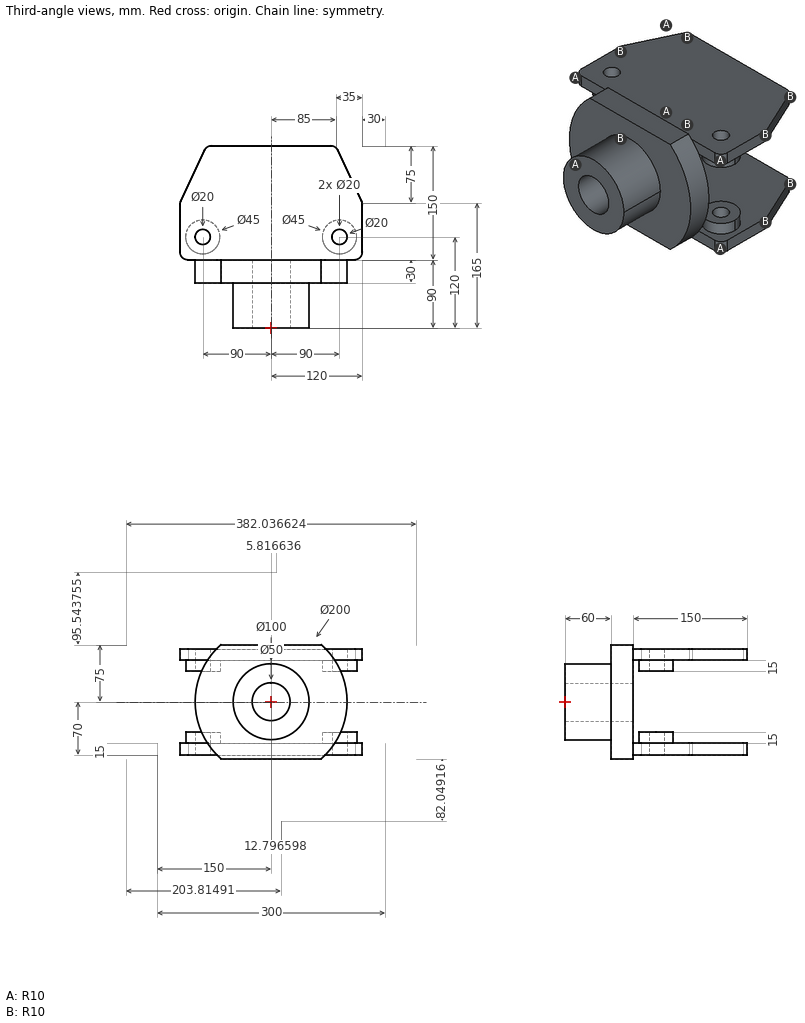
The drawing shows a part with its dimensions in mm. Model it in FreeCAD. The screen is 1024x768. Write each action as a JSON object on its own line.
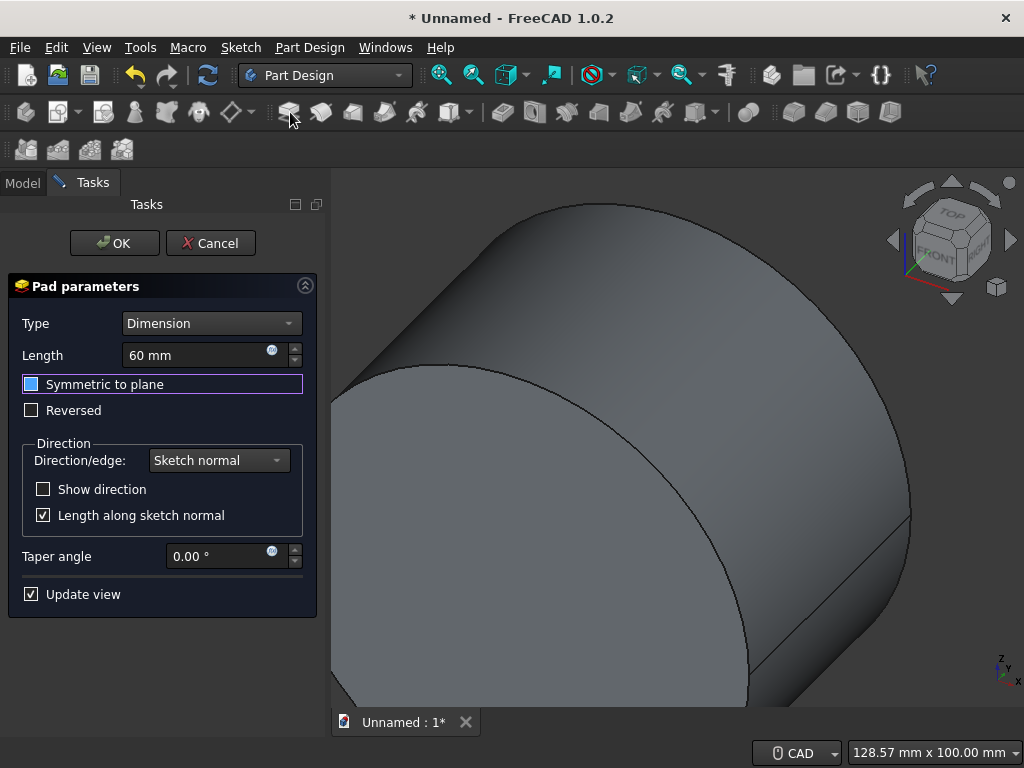
{"action": "left_click", "coordinate": [30, 410]}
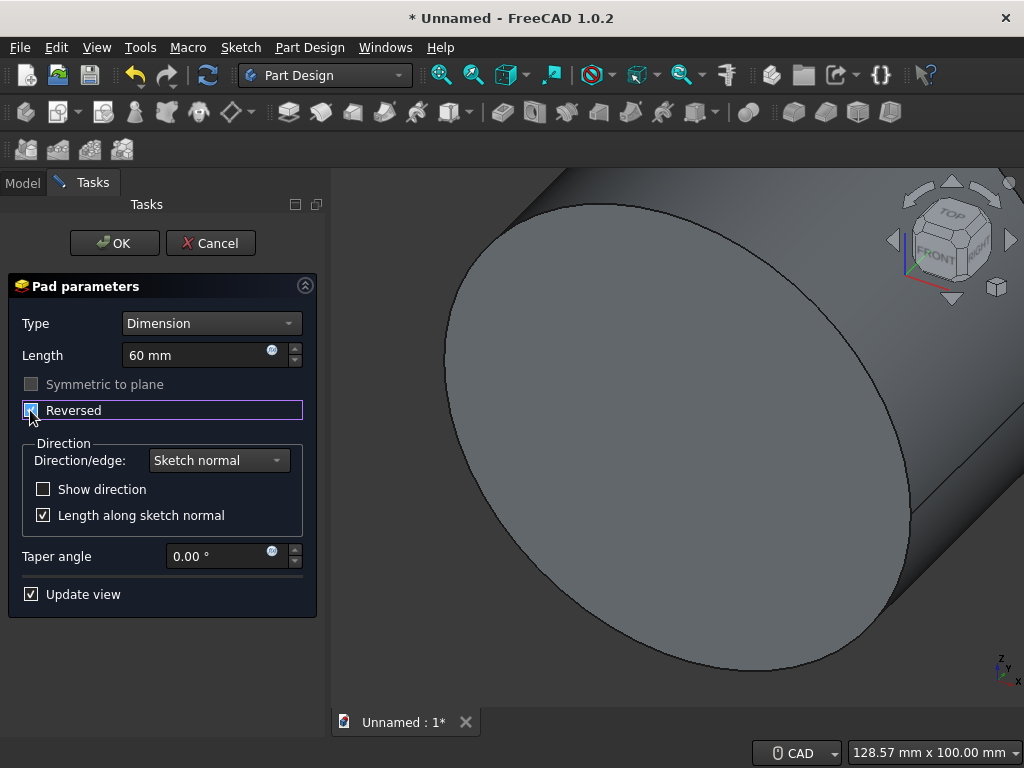
{"action": "left_click", "coordinate": [115, 243]}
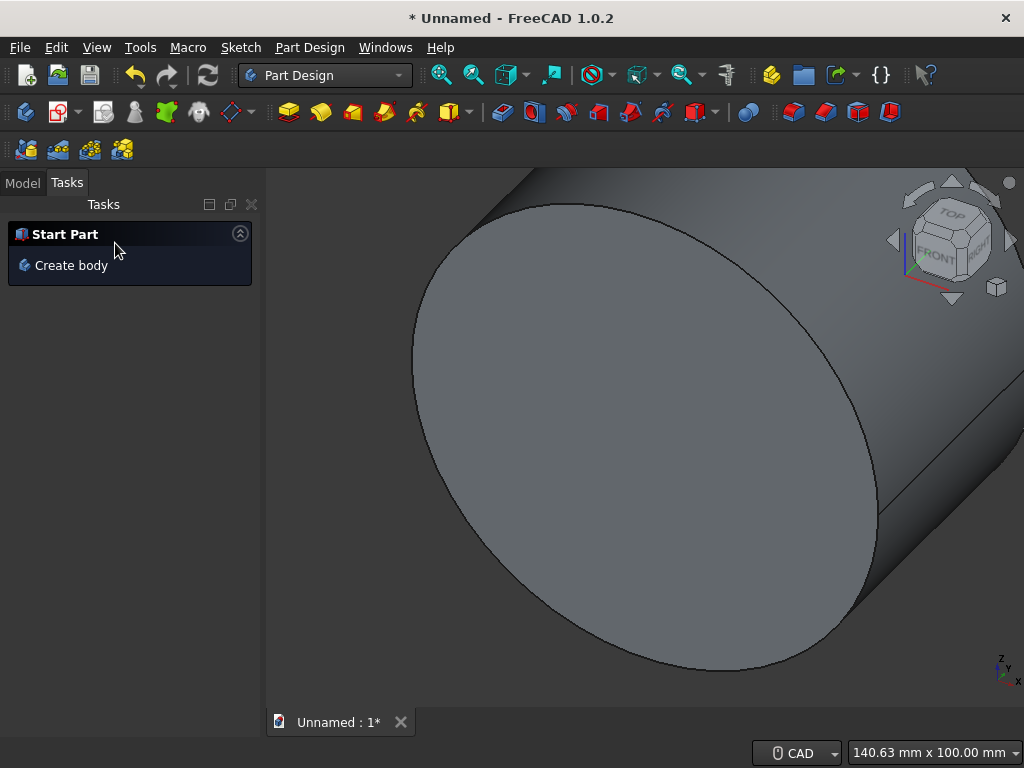
{"action": "left_click", "coordinate": [442, 76]}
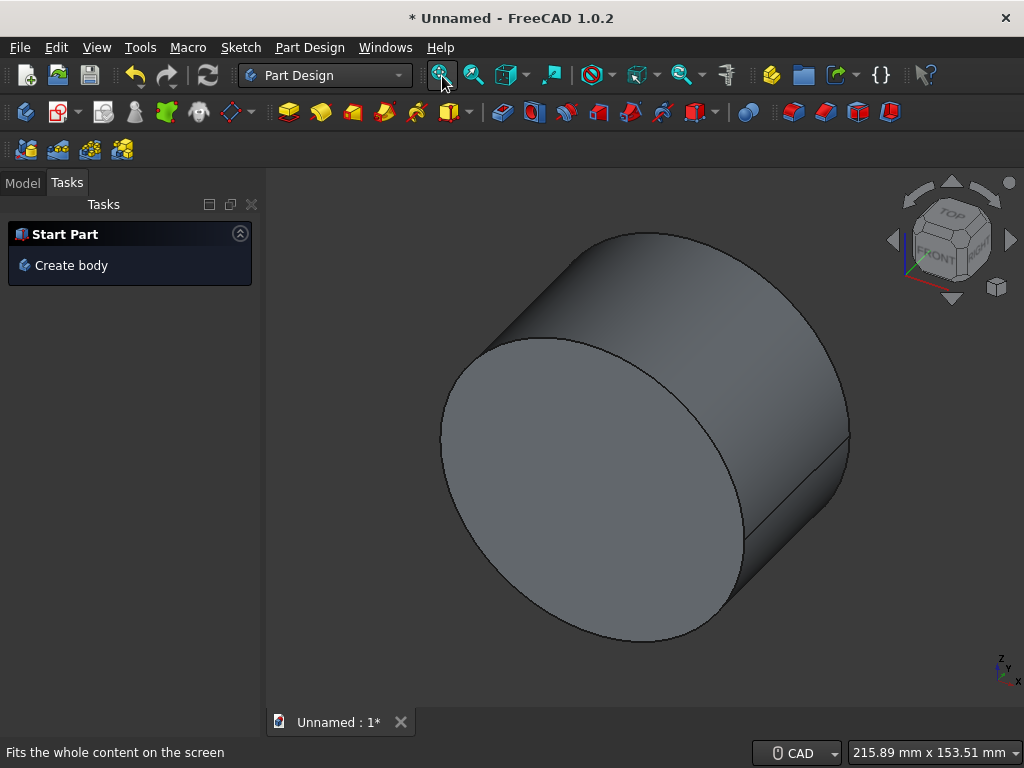
{"action": "key", "text": "4"}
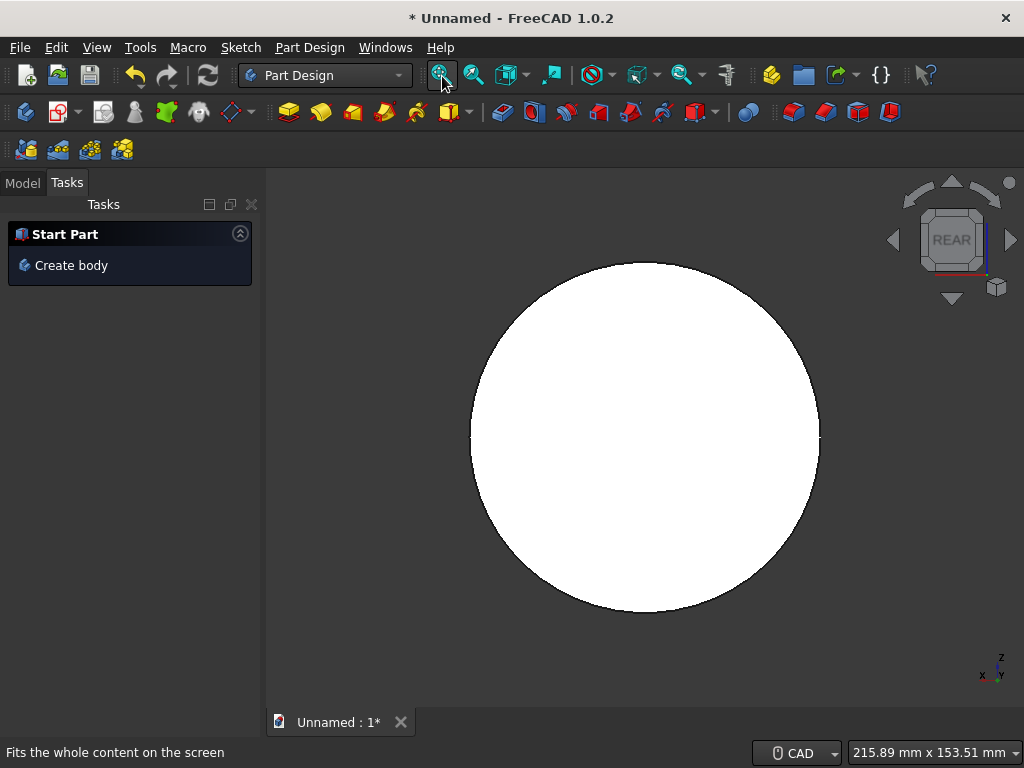
{"action": "left_click", "coordinate": [645, 437]}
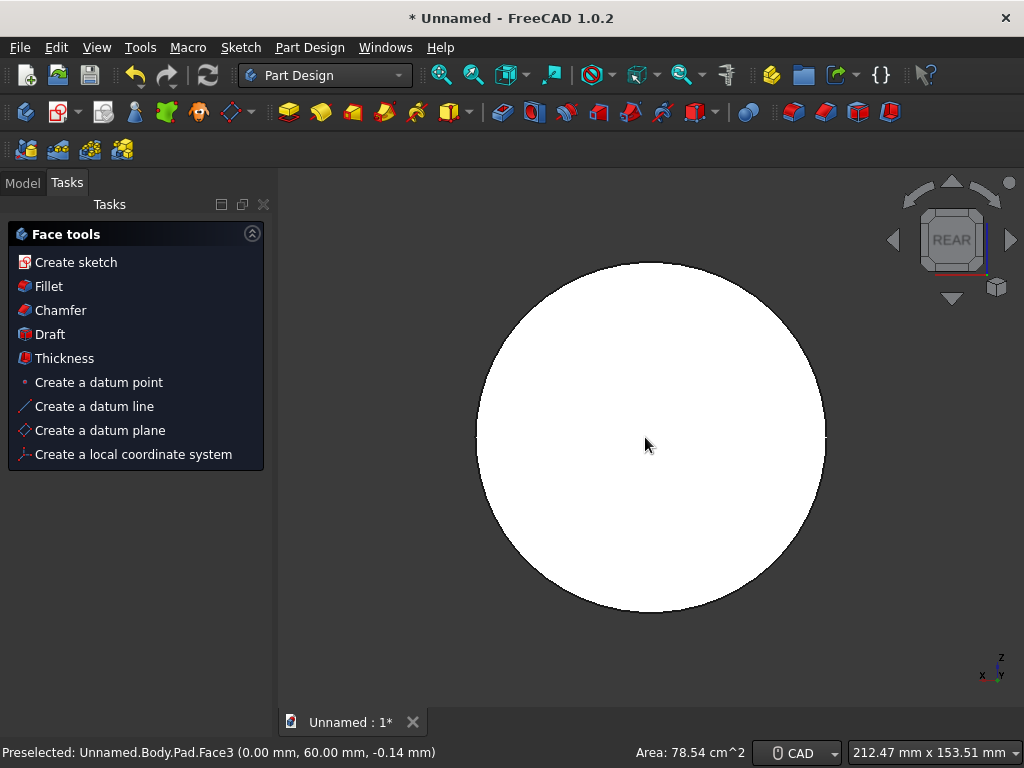
{"action": "left_click", "coordinate": [58, 112]}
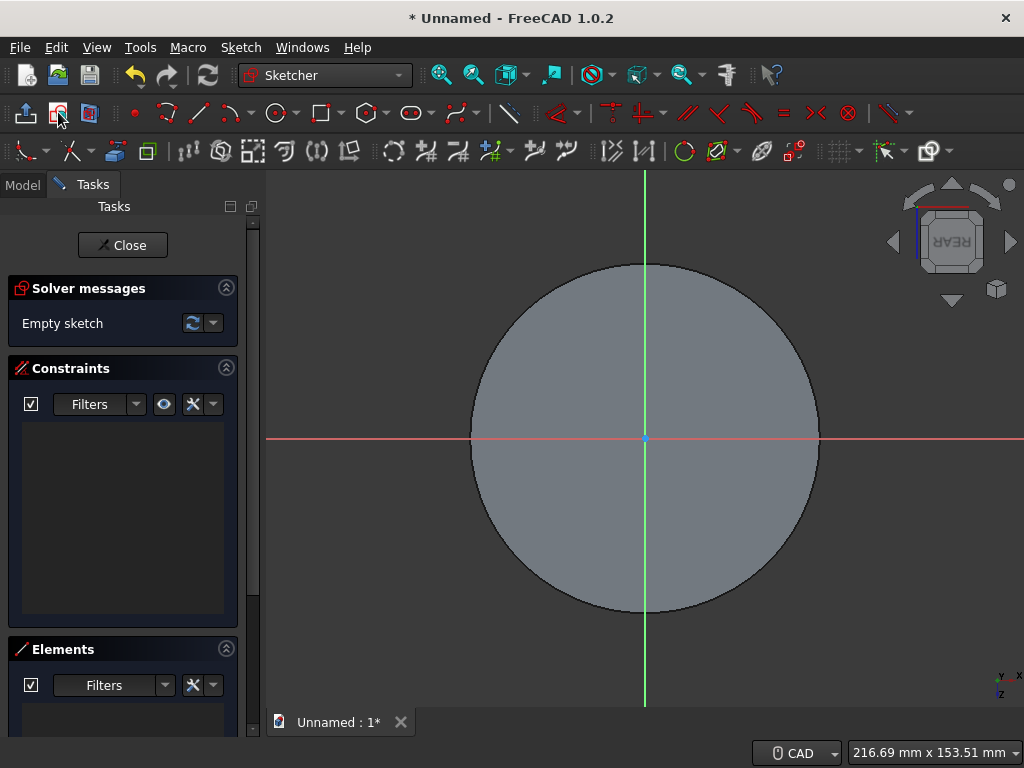
{"action": "scroll", "coordinate": [521, 438], "scroll_direction": "down", "scroll_amount": 4}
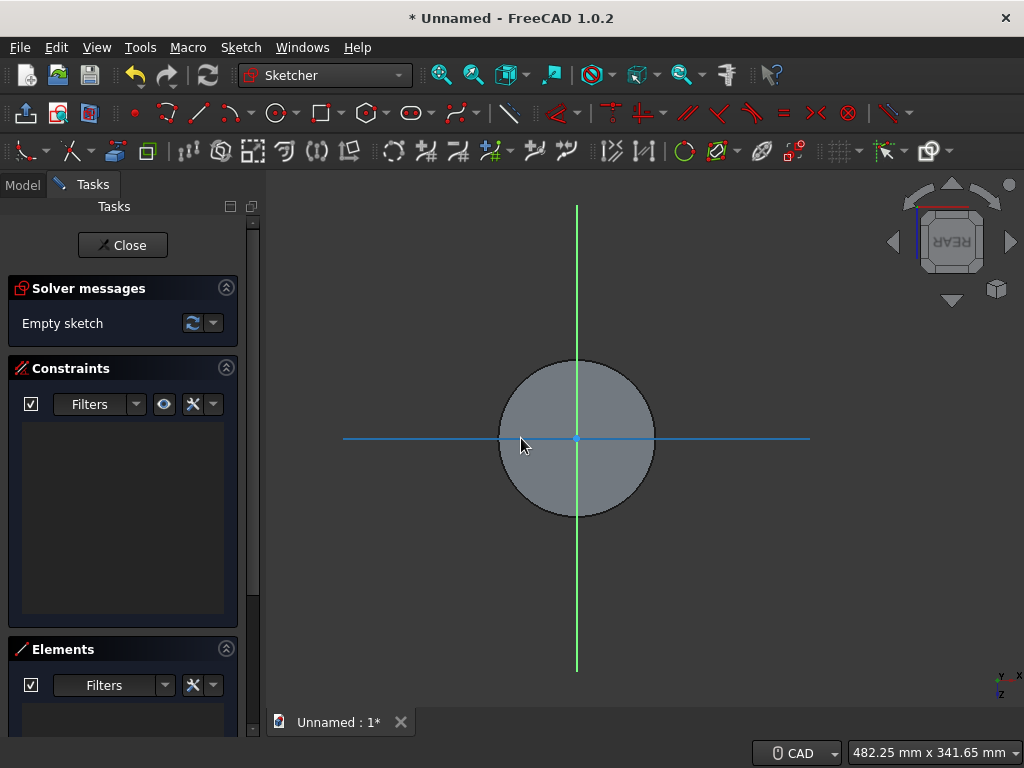
{"action": "key", "text": "g c"}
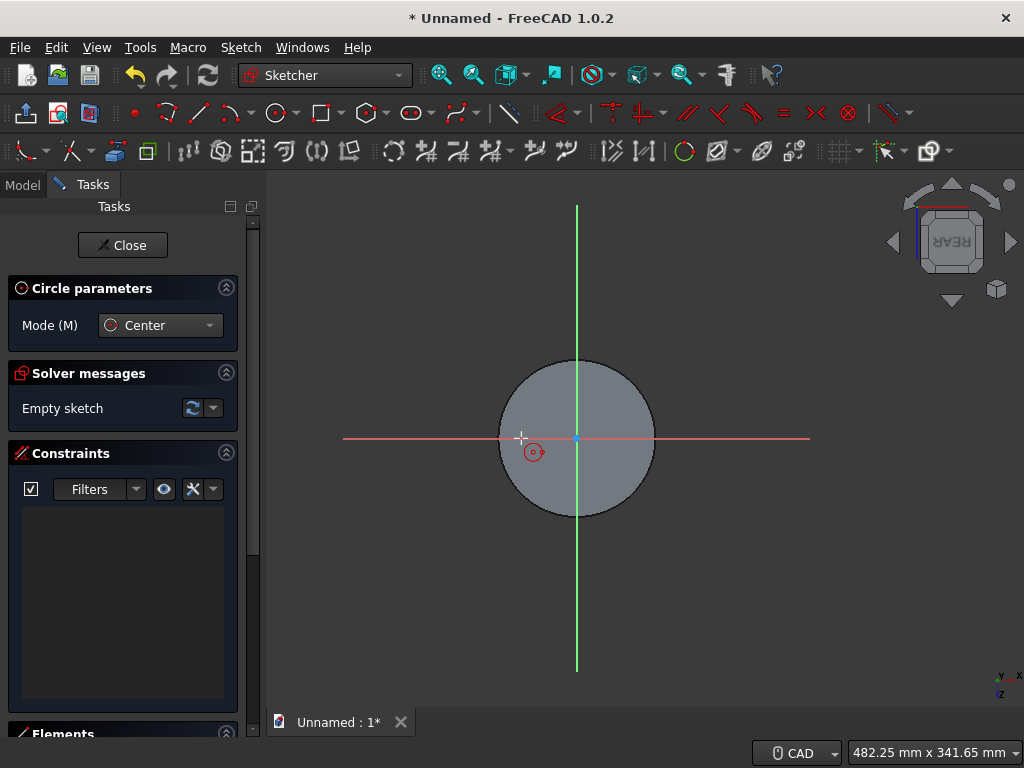
{"action": "left_click", "coordinate": [577, 439]}
{"action": "left_click", "coordinate": [688, 327]}
{"action": "key", "text": "Escape"}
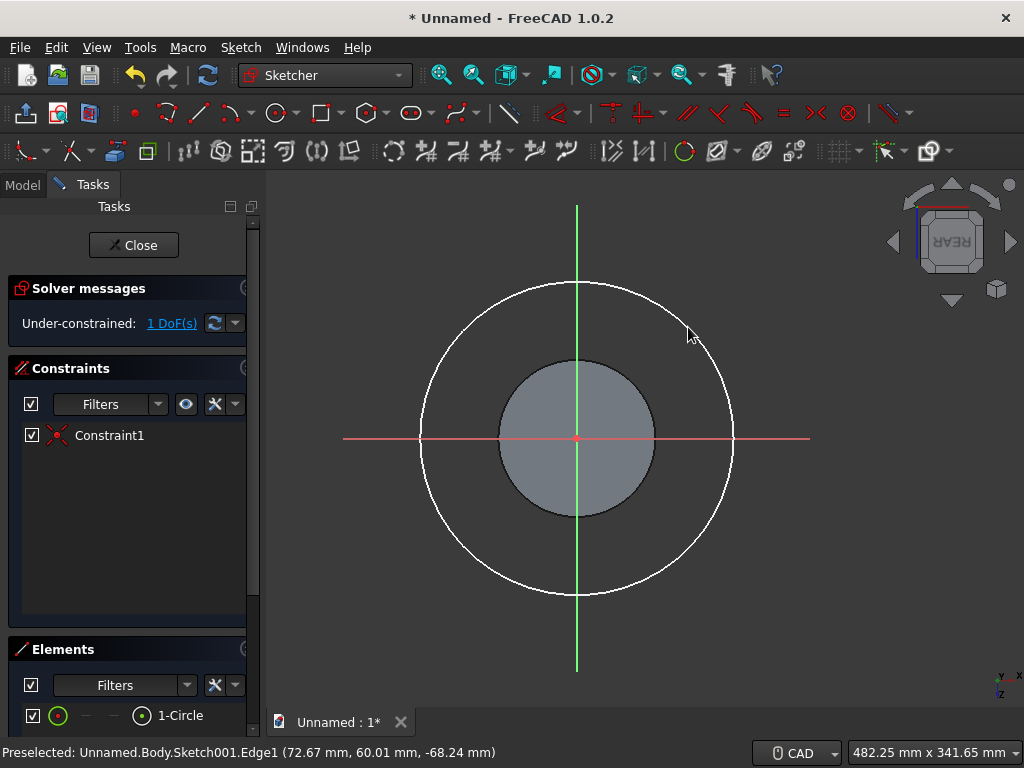
{"action": "key", "text": "d"}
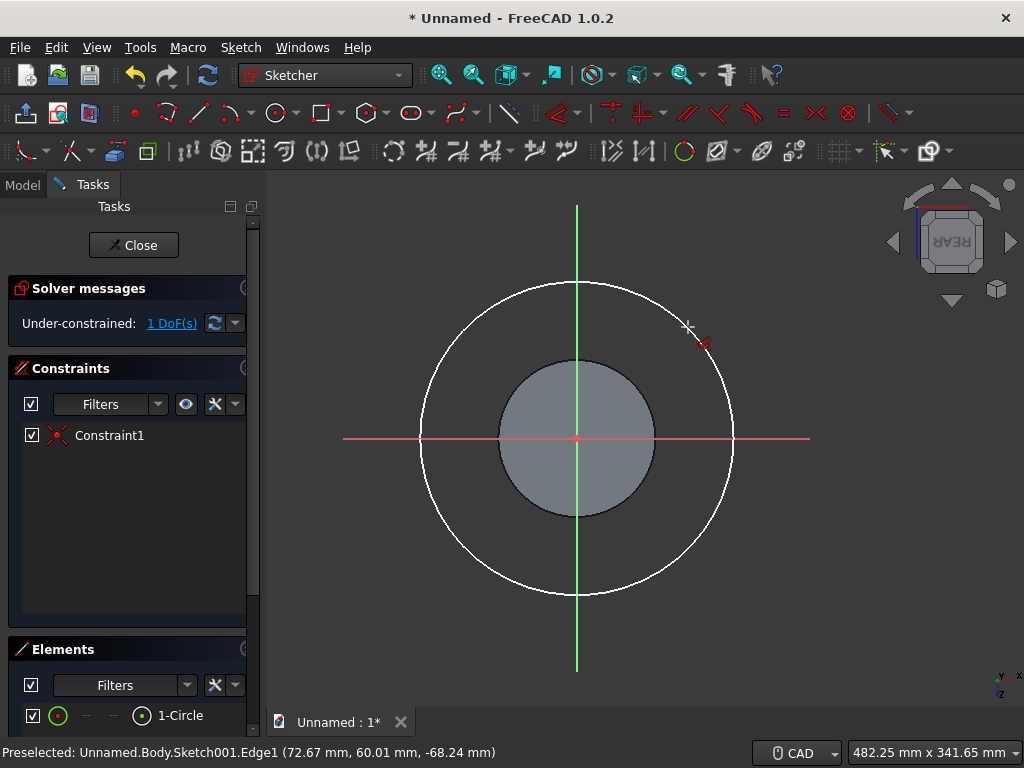
{"action": "left_click", "coordinate": [687, 327]}
{"action": "left_click", "coordinate": [709, 304]}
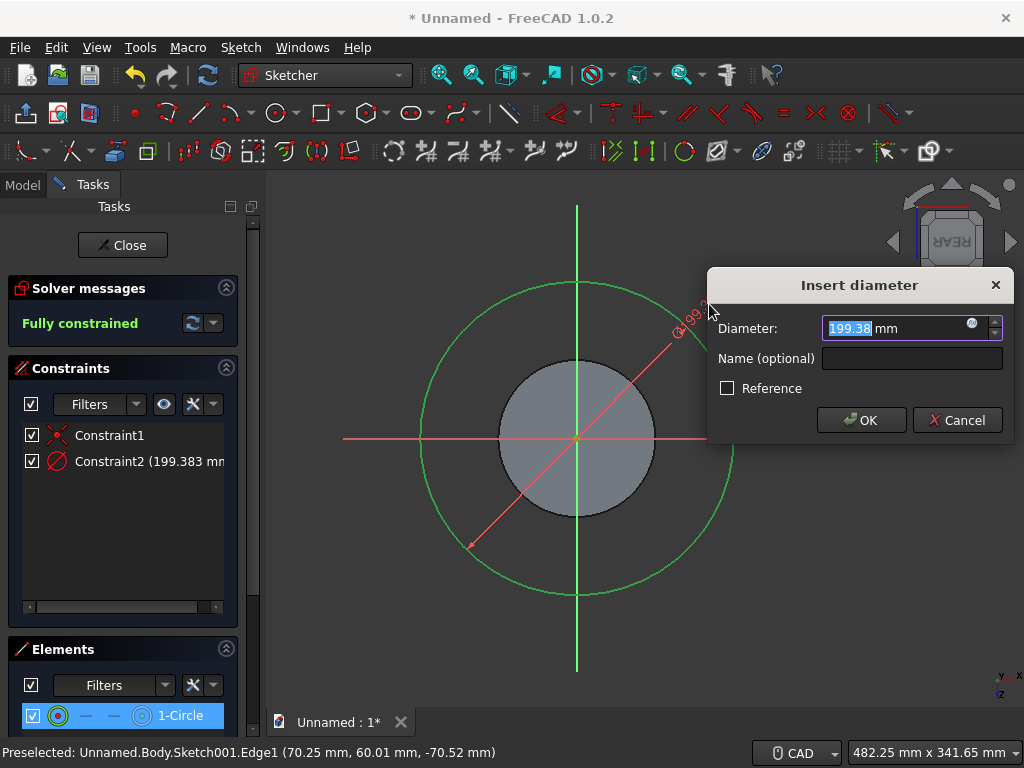
{"action": "type", "text": "200"}
{"action": "key", "text": "Return"}
{"action": "key", "text": "Escape"}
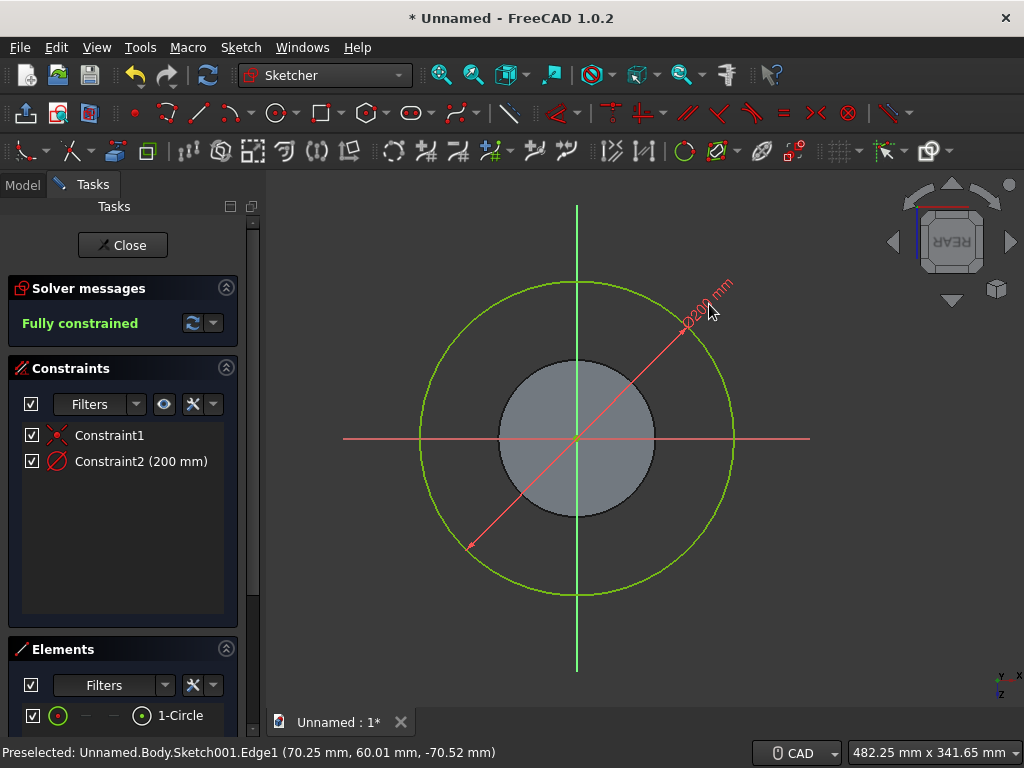
{"action": "left_click", "coordinate": [123, 245]}